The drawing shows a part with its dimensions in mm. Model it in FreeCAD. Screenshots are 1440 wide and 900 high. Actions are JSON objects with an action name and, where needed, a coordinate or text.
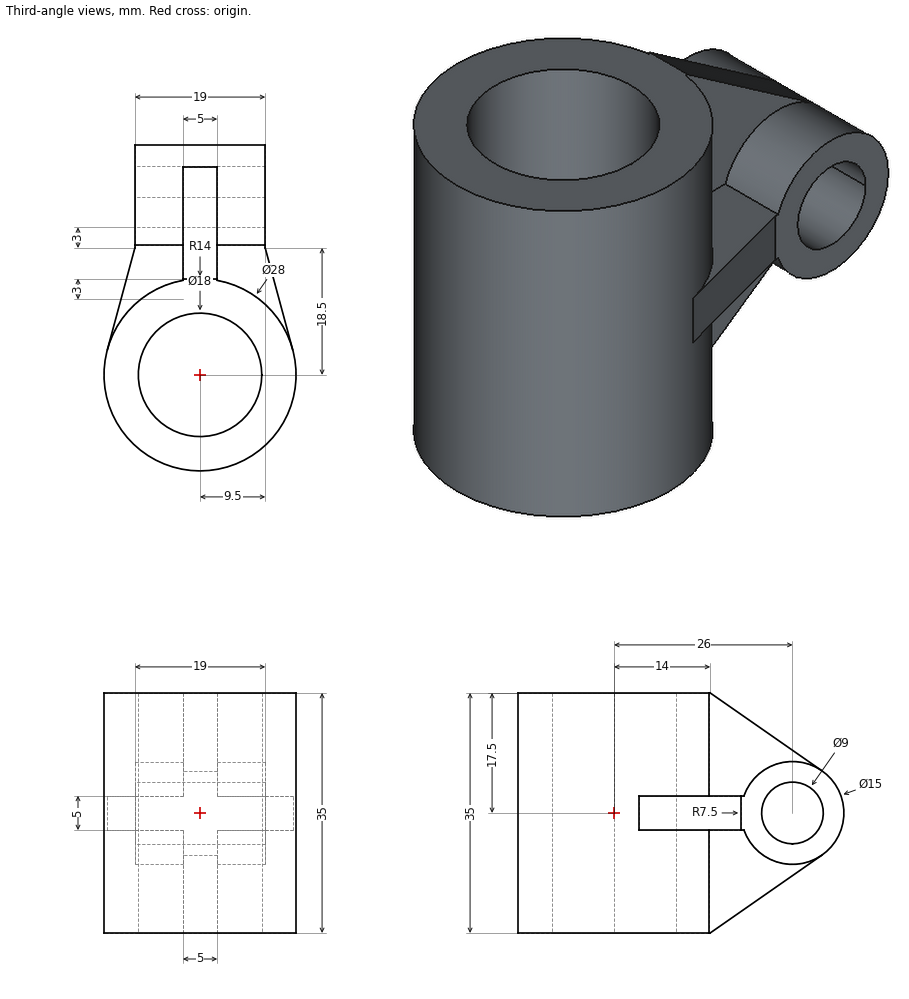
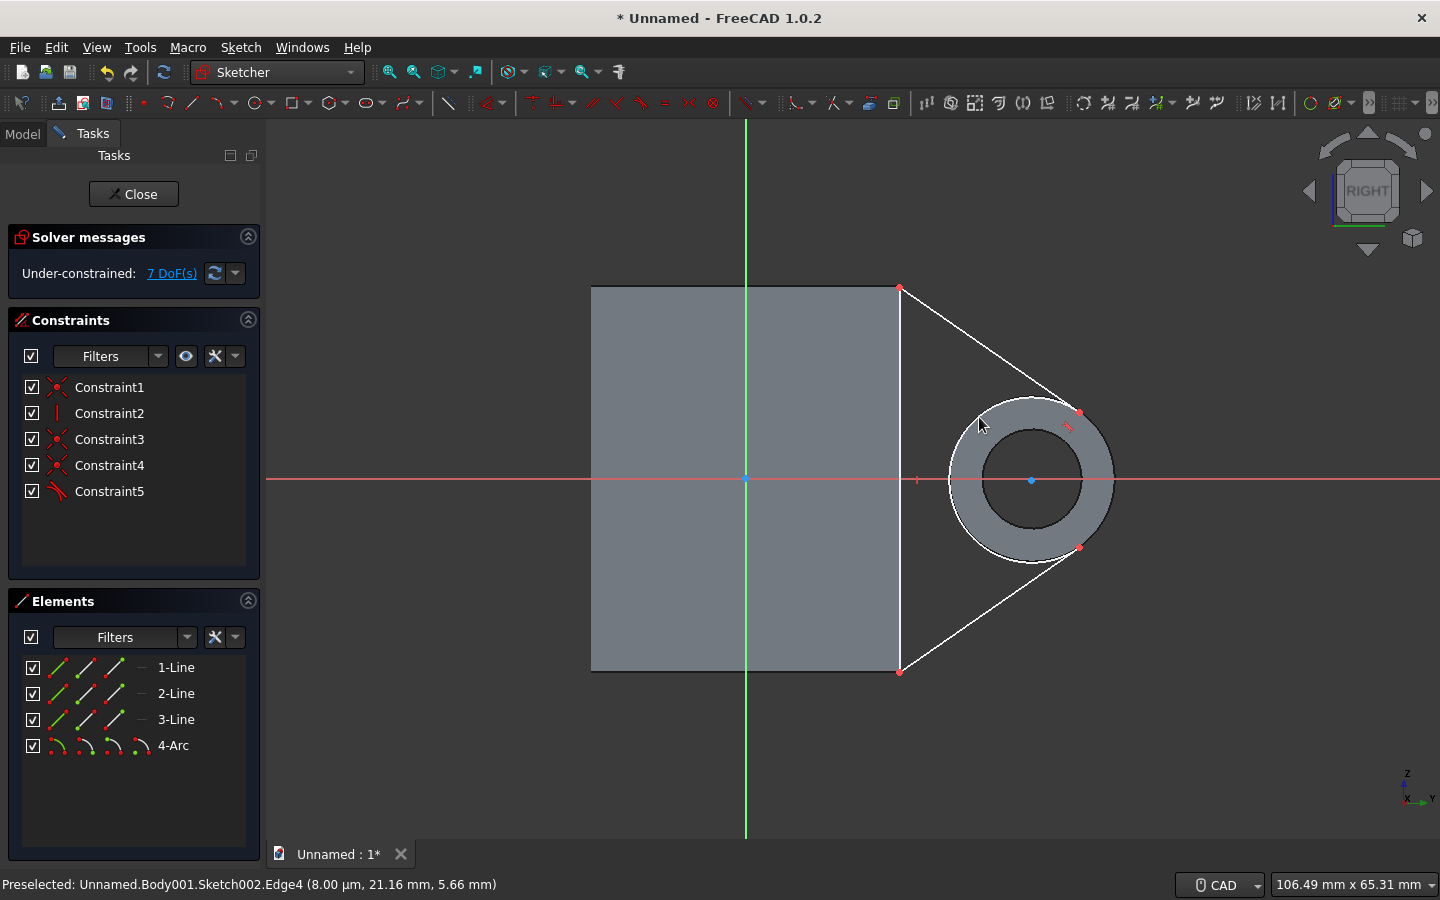
{"action": "left_click", "coordinate": [954, 635]}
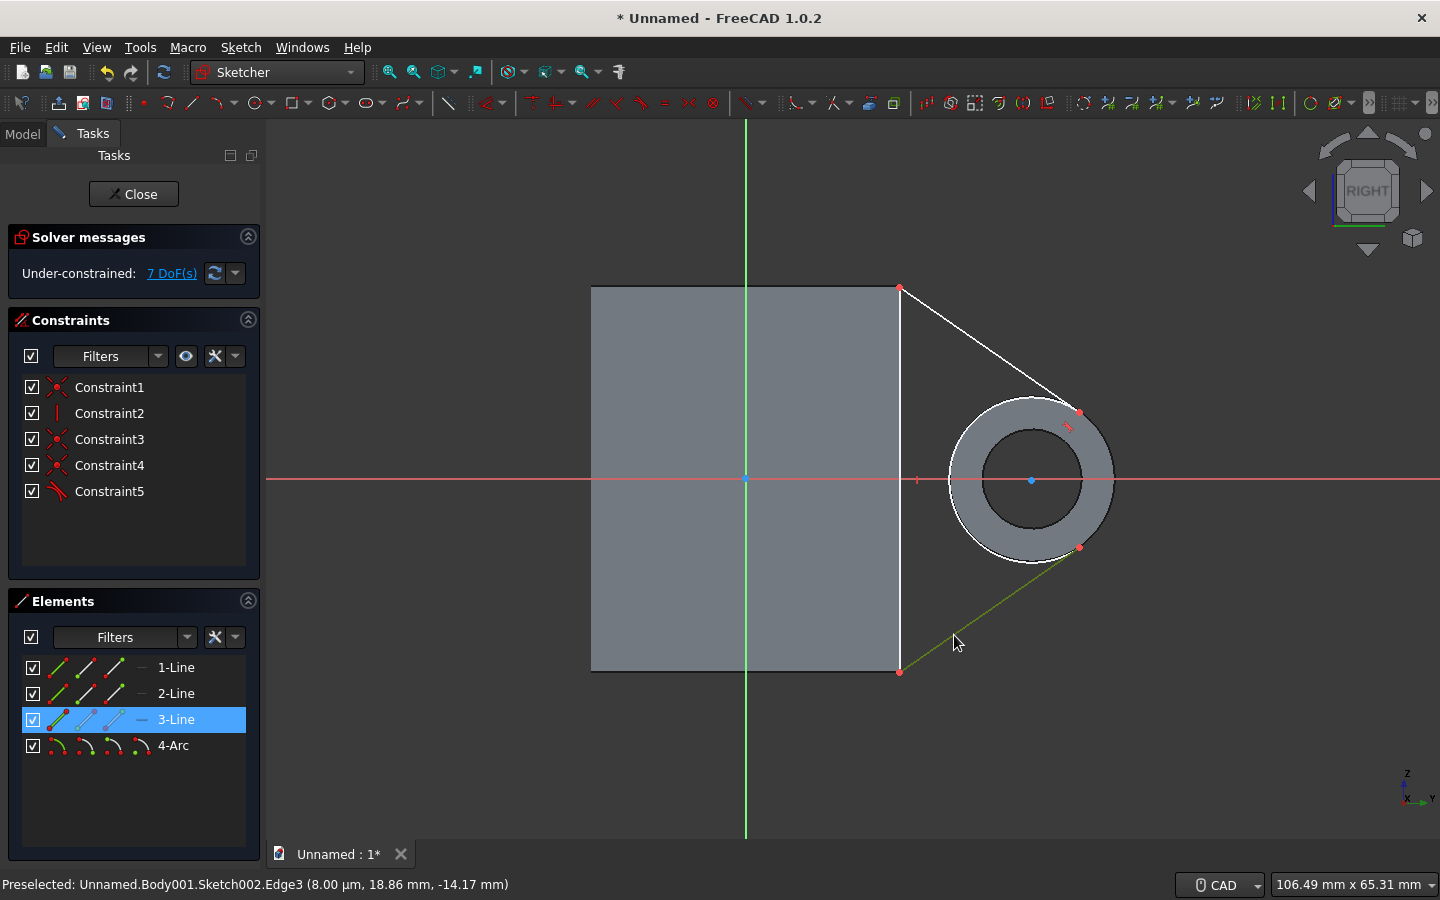
{"action": "left_click", "coordinate": [979, 417]}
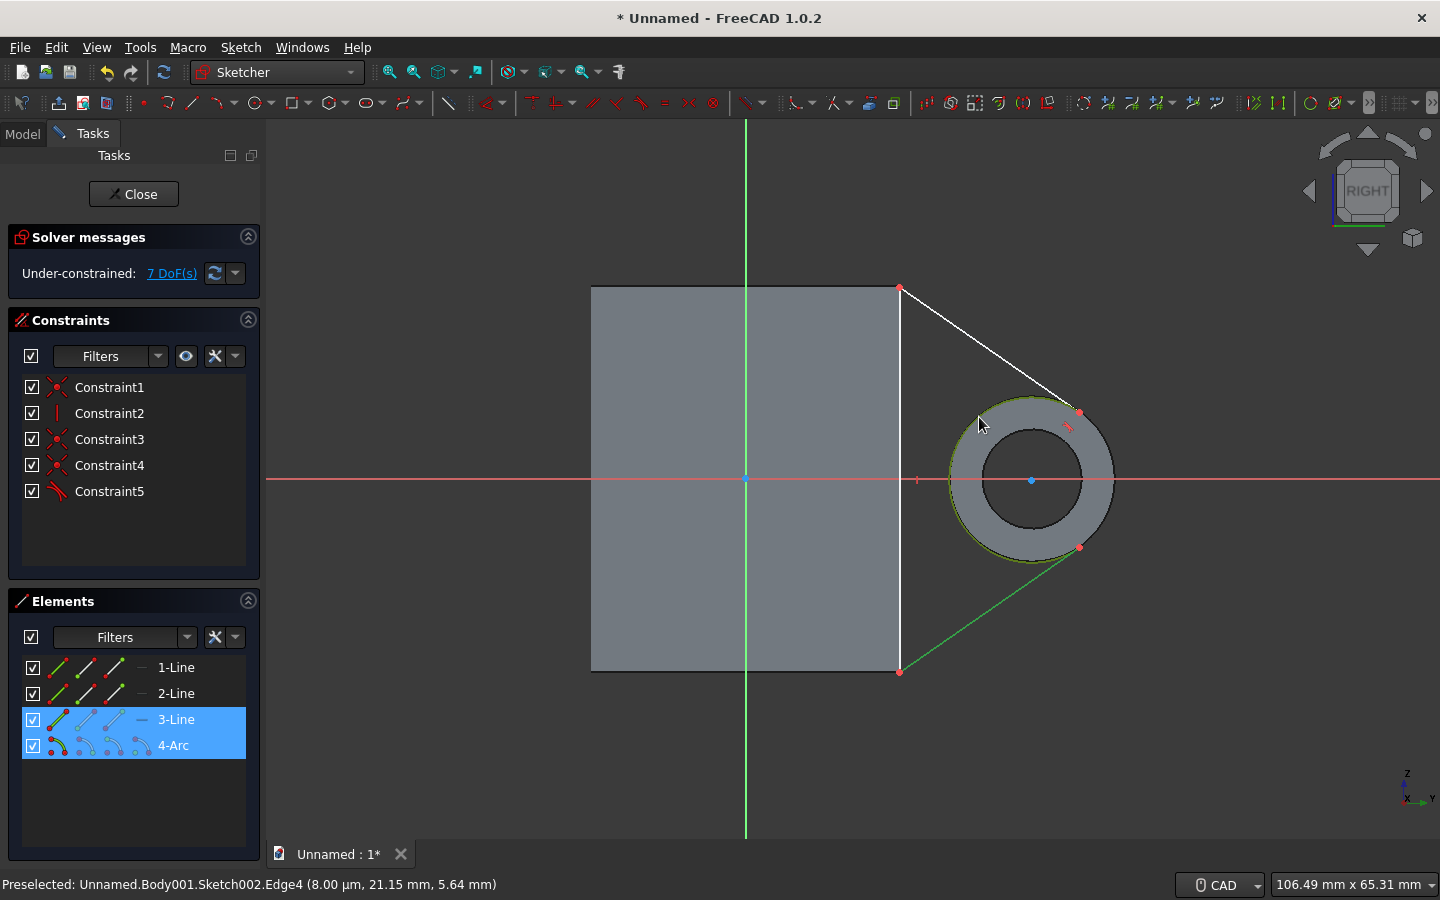
{"action": "key", "text": "t"}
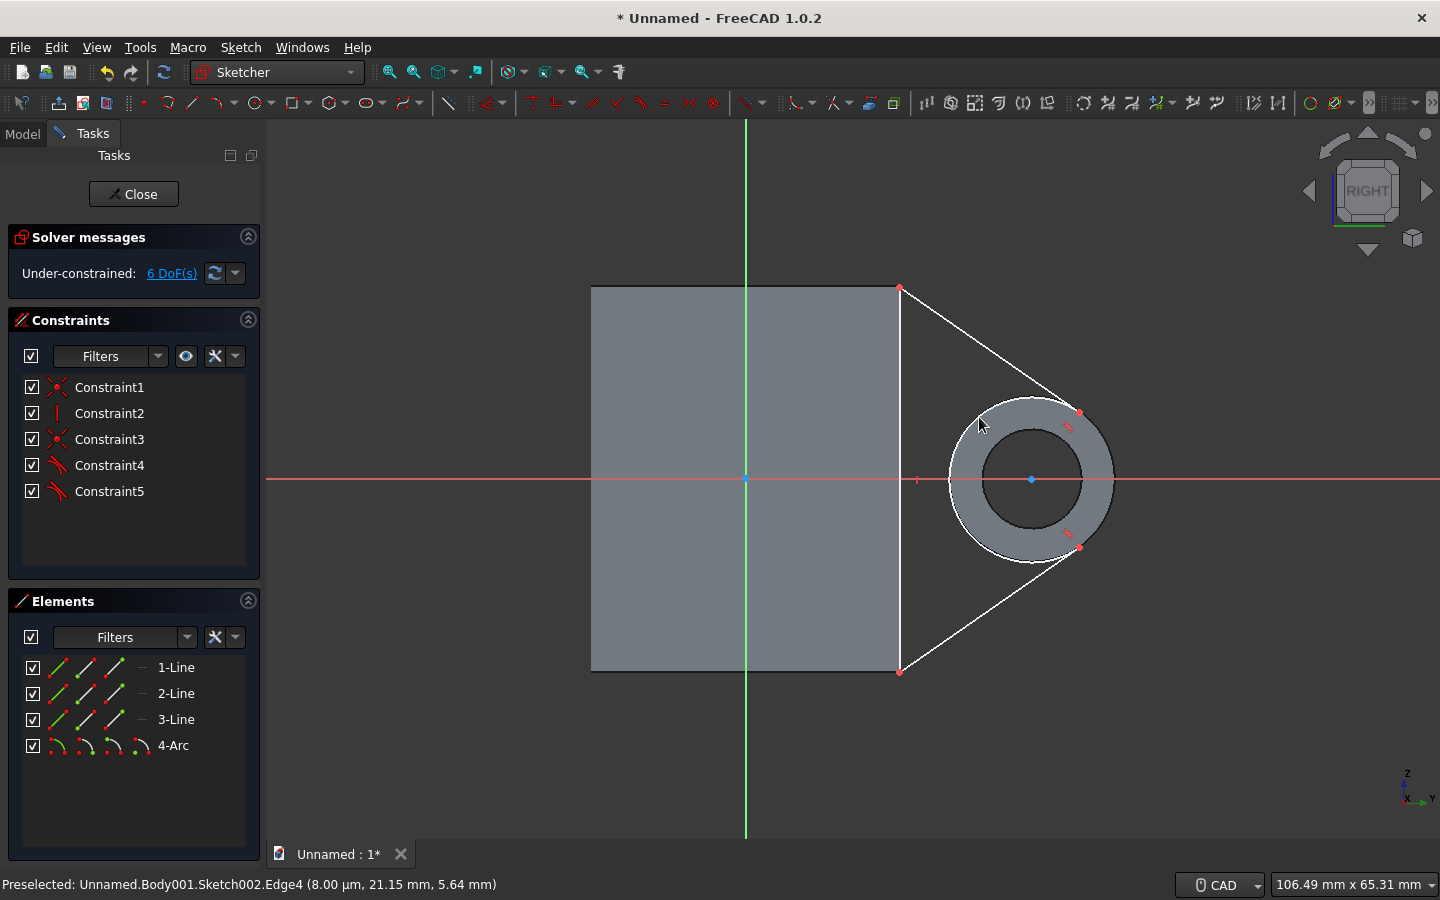
{"action": "left_click", "coordinate": [1032, 480]}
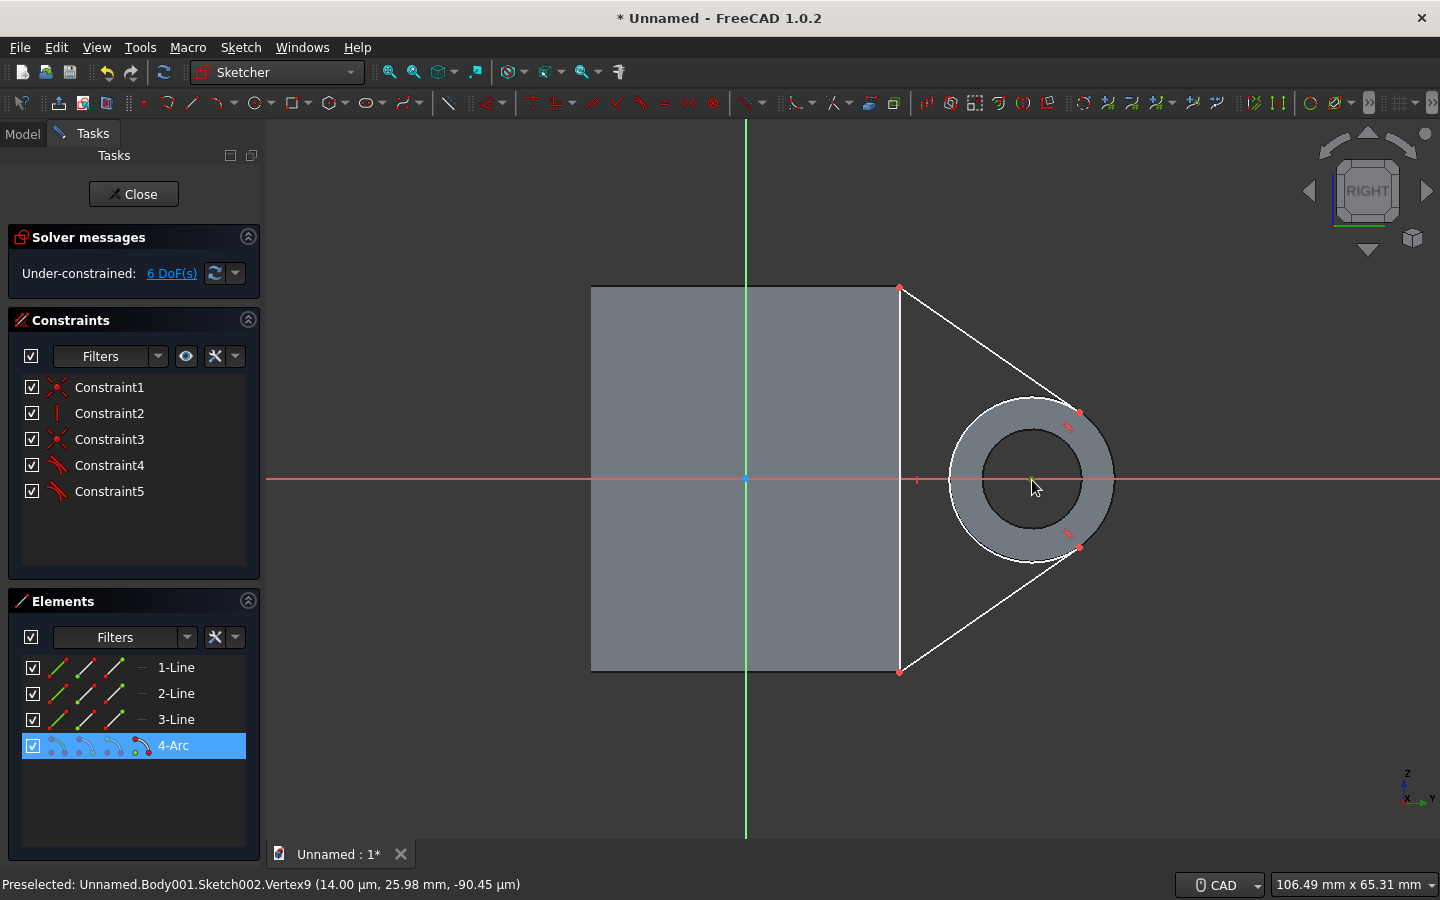
{"action": "left_click", "coordinate": [364, 479]}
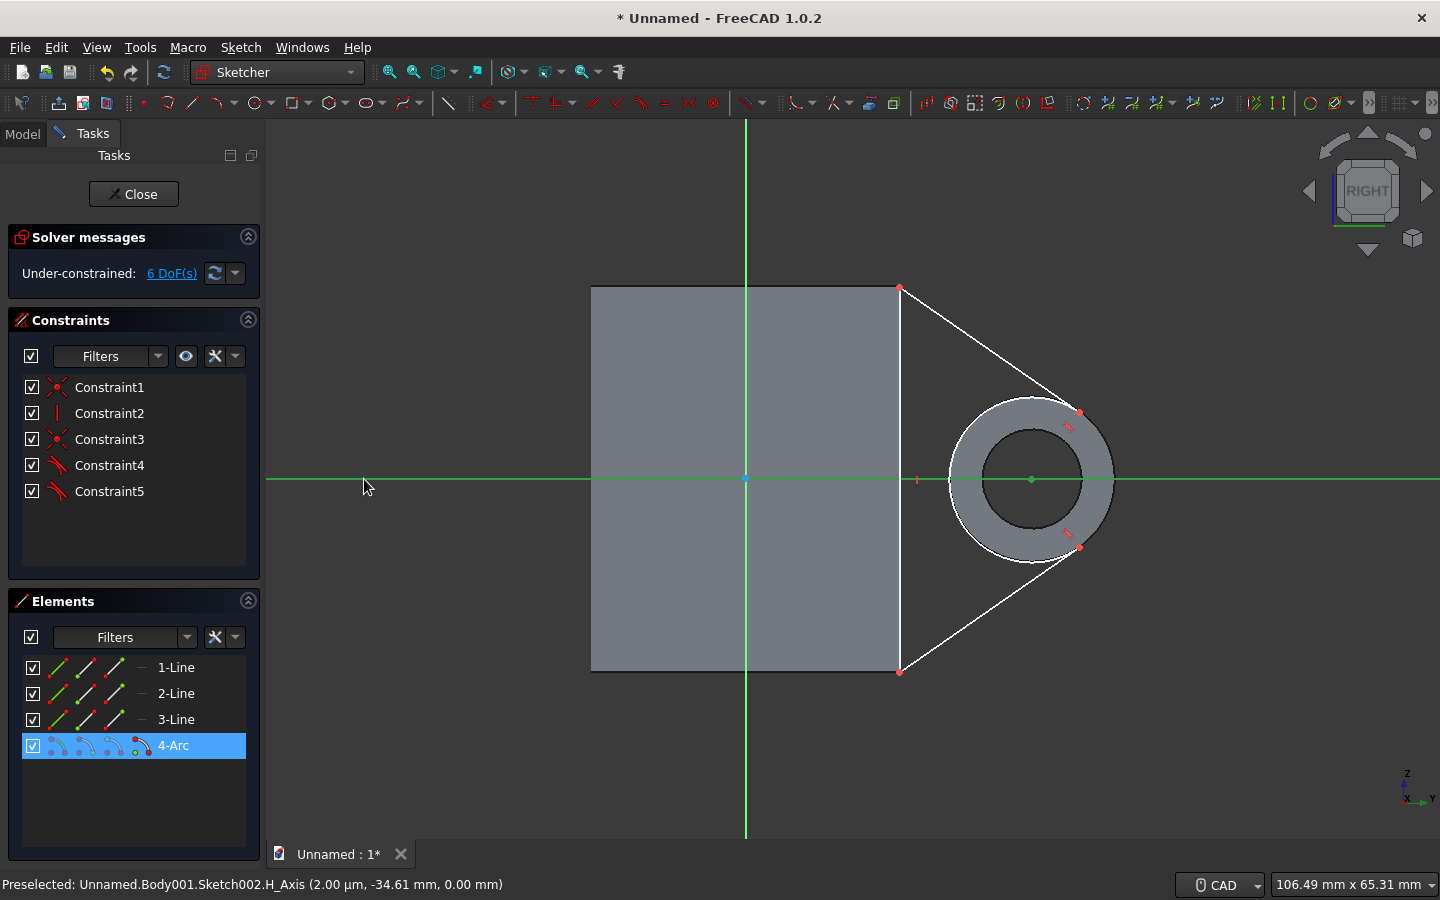
{"action": "key", "text": "c"}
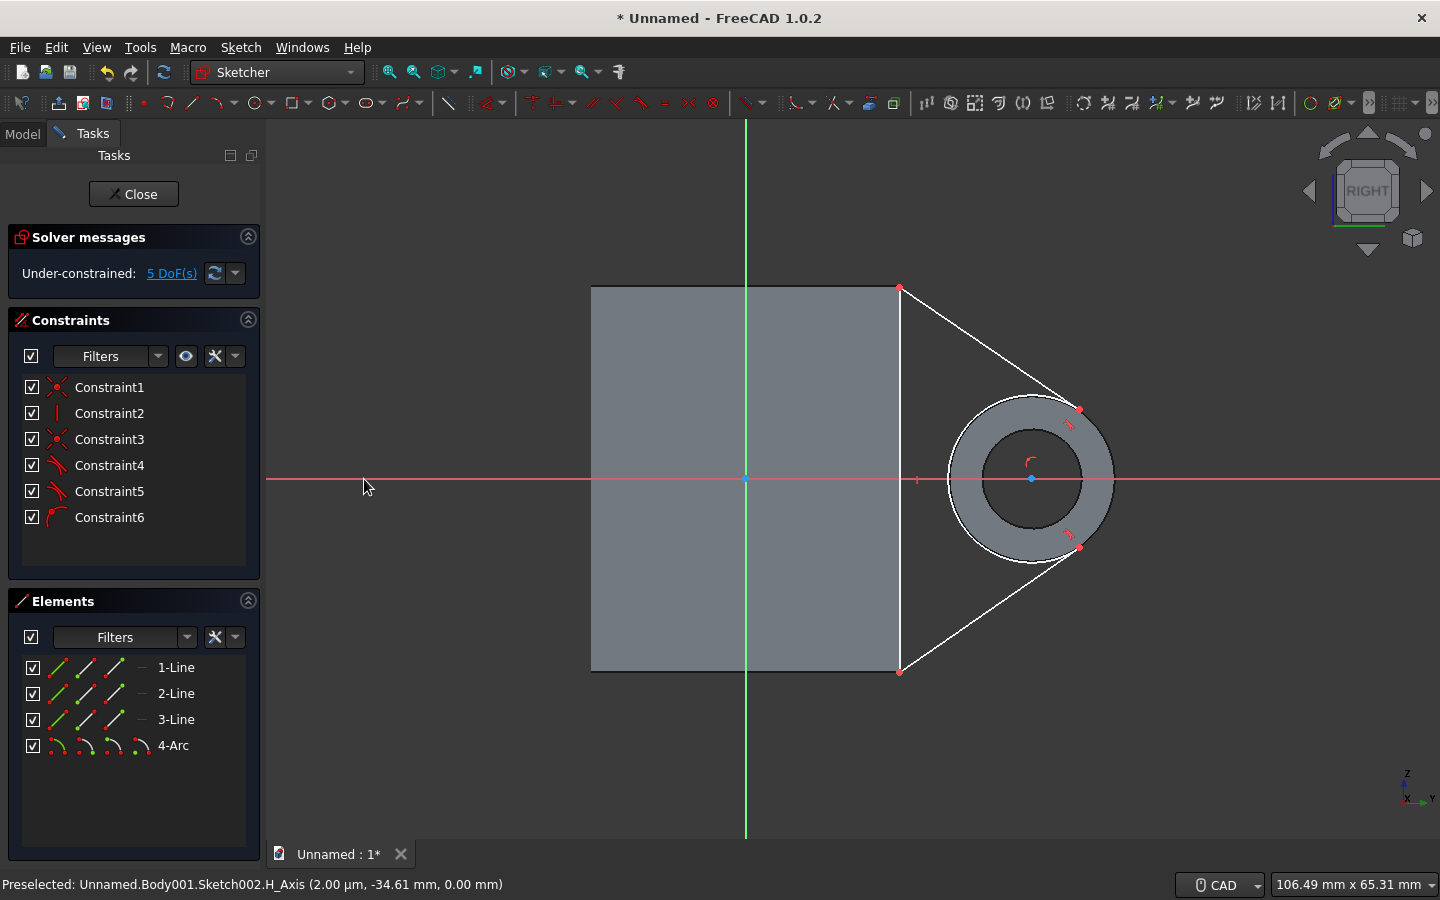
{"action": "key", "text": "d"}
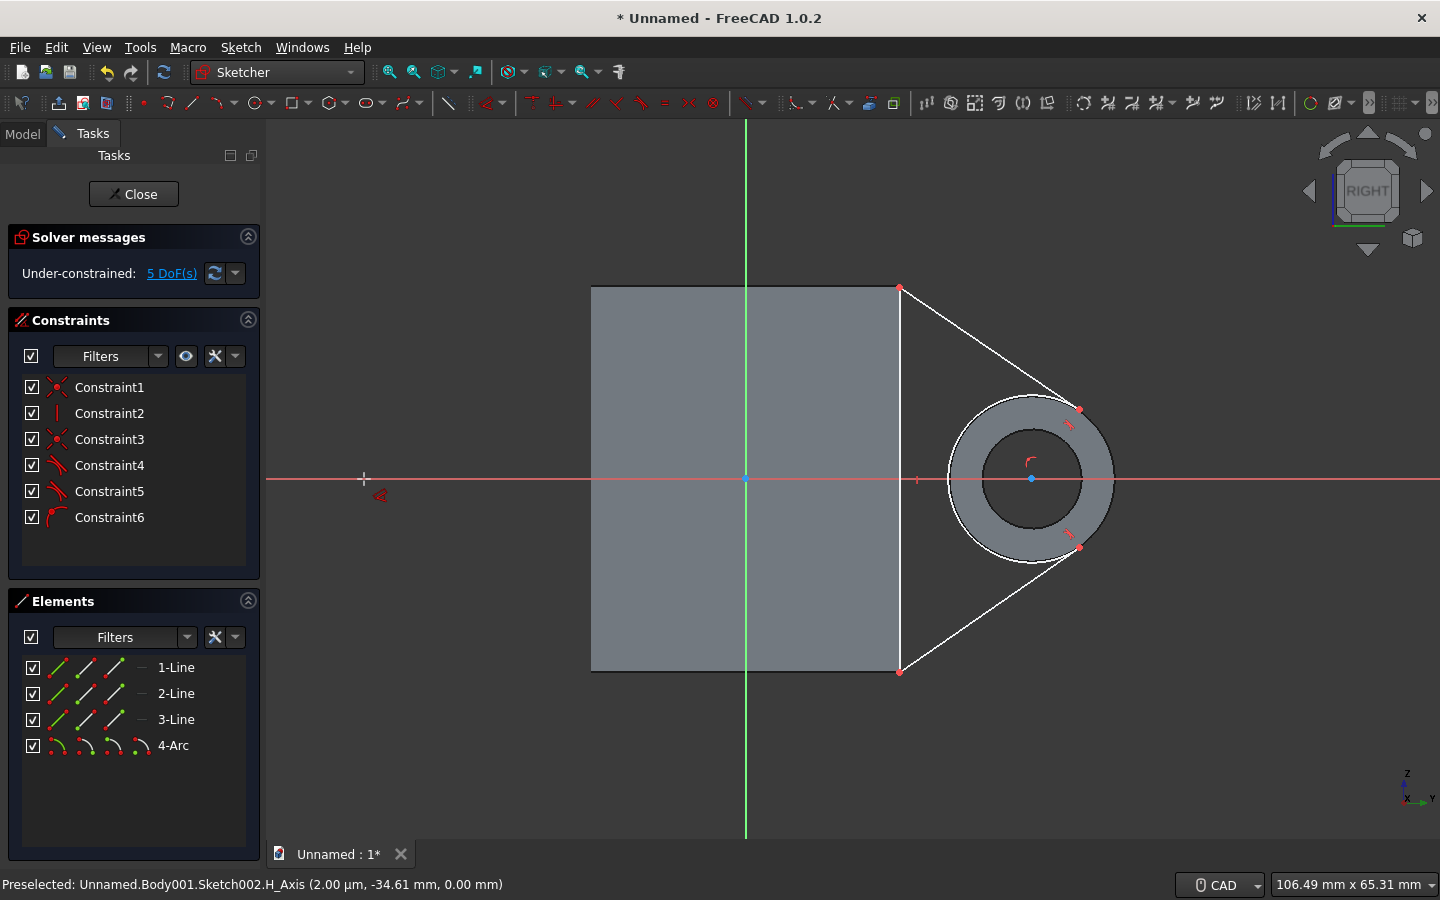
{"action": "left_click", "coordinate": [978, 415]}
{"action": "left_click", "coordinate": [957, 391]}